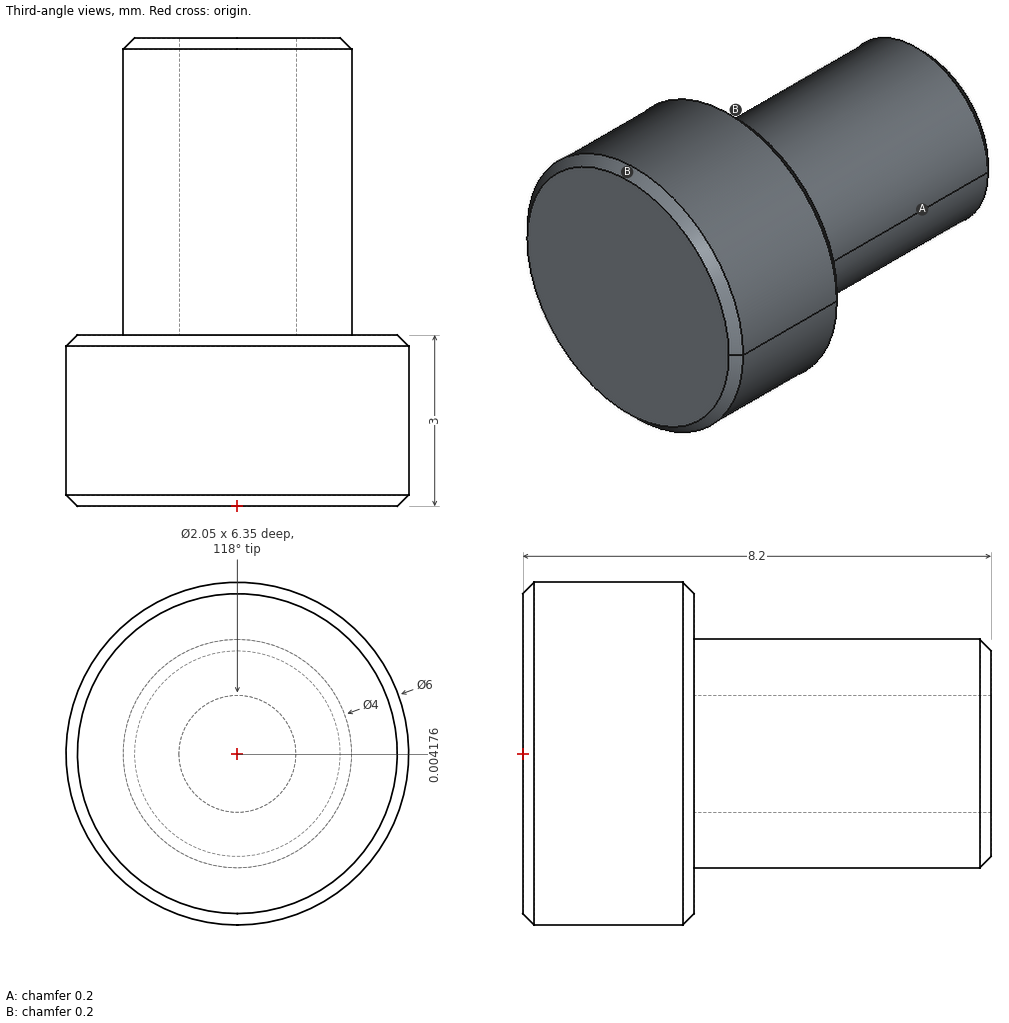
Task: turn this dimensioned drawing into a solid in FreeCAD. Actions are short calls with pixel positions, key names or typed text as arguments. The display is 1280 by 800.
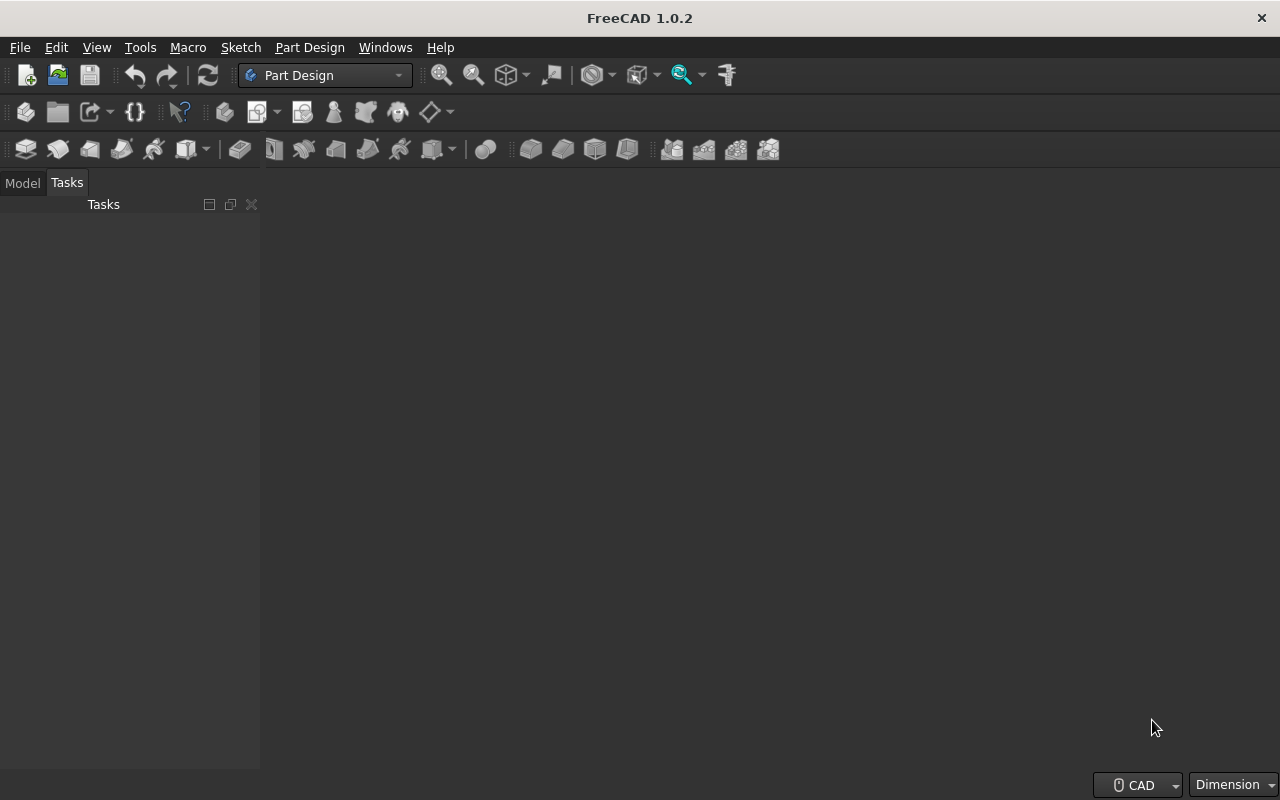
click(26, 76)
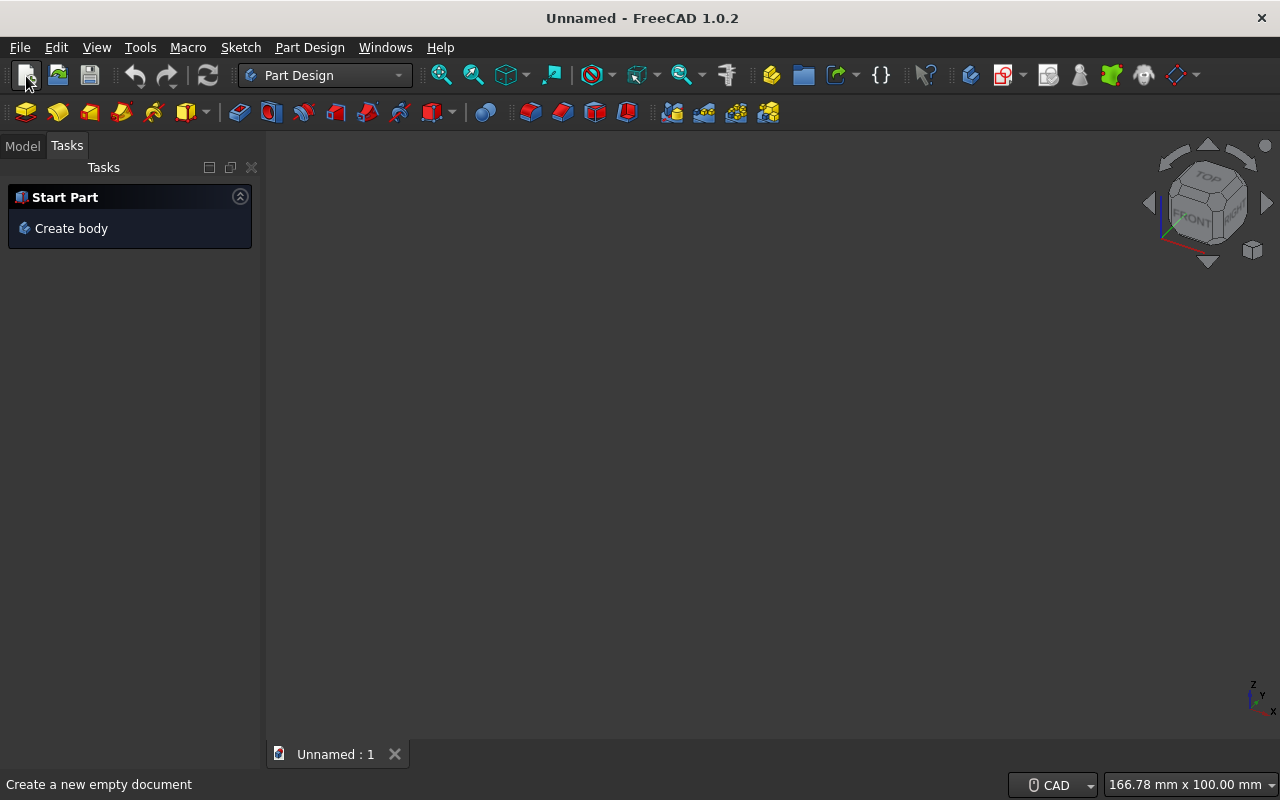
click(1004, 76)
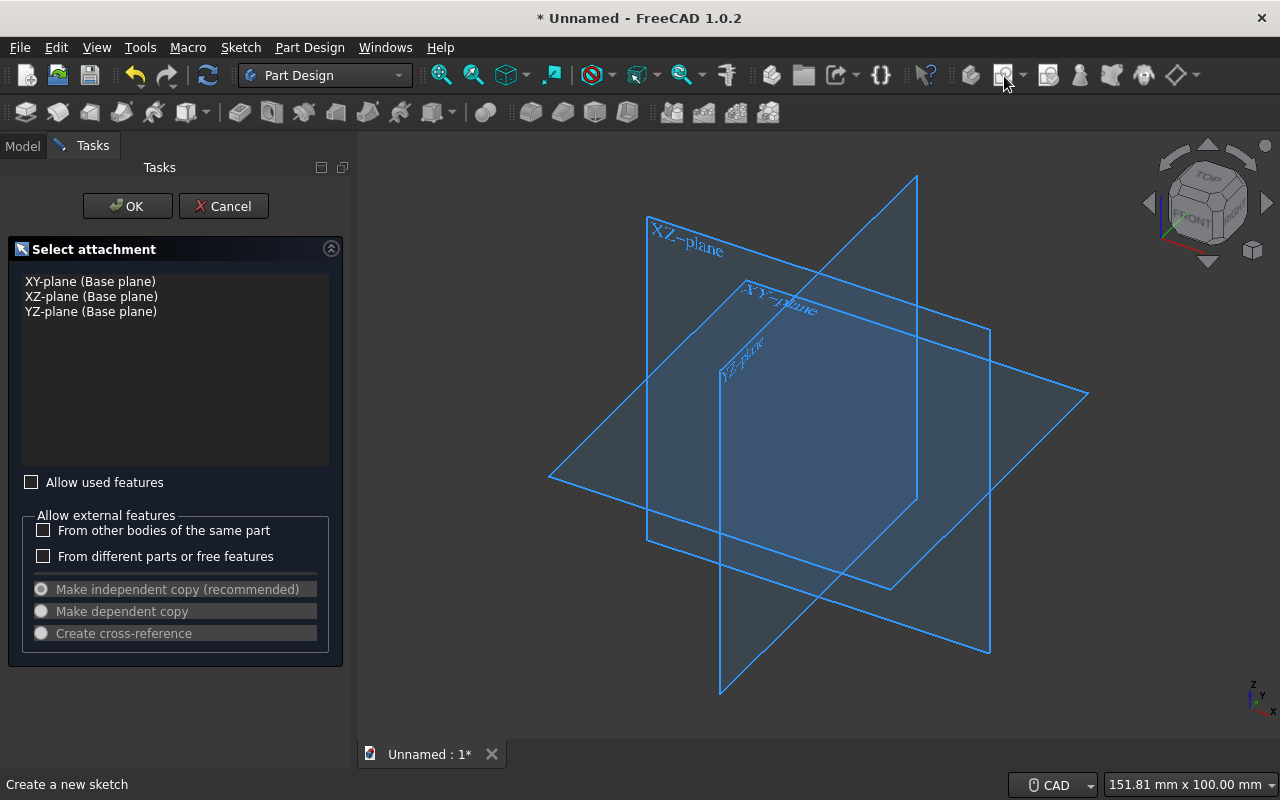
click(82, 296)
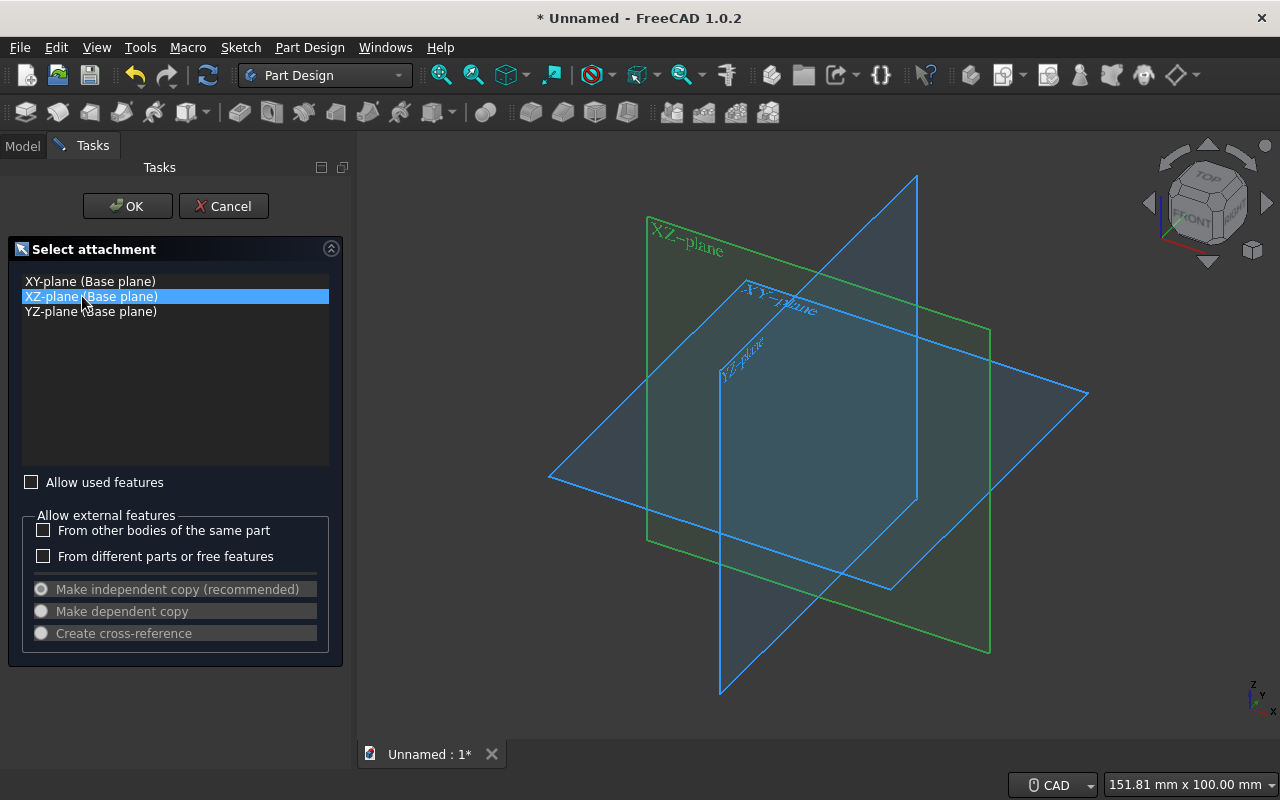
click(128, 206)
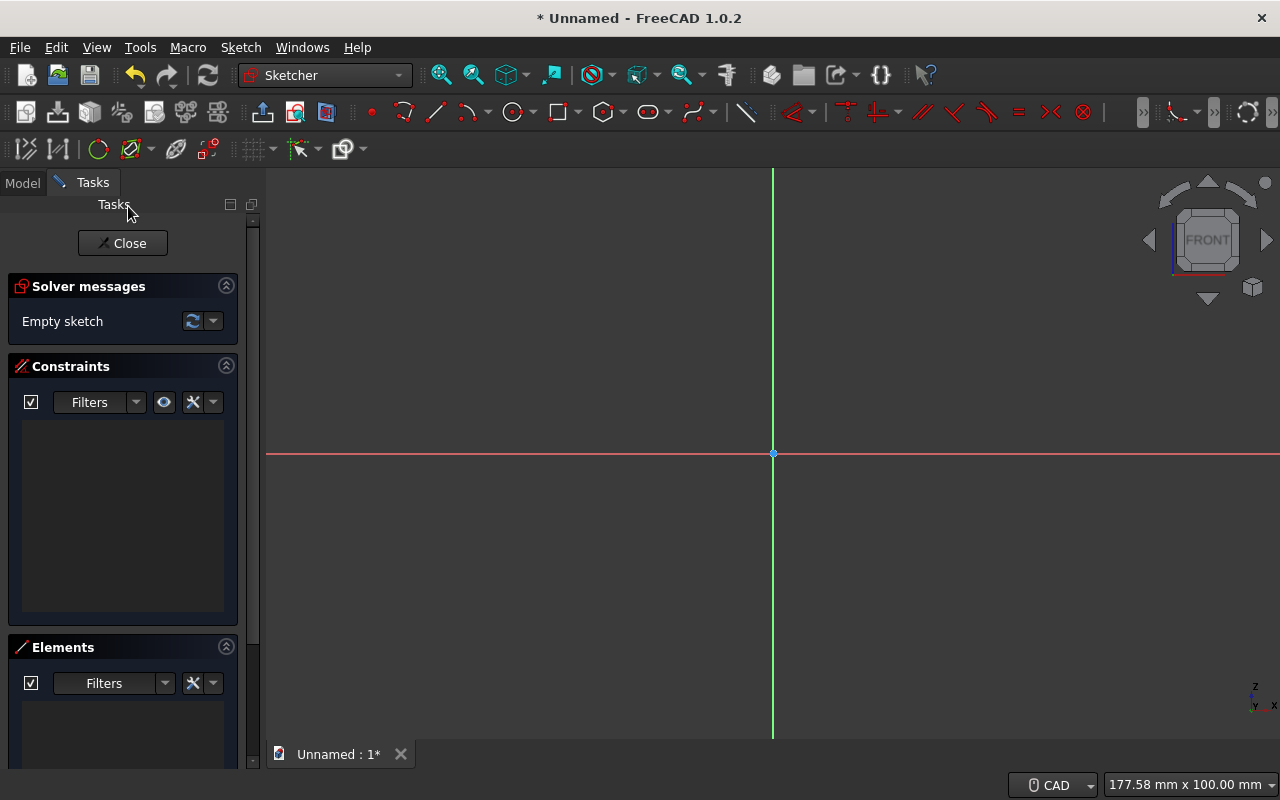
scroll(777, 454, up, 14)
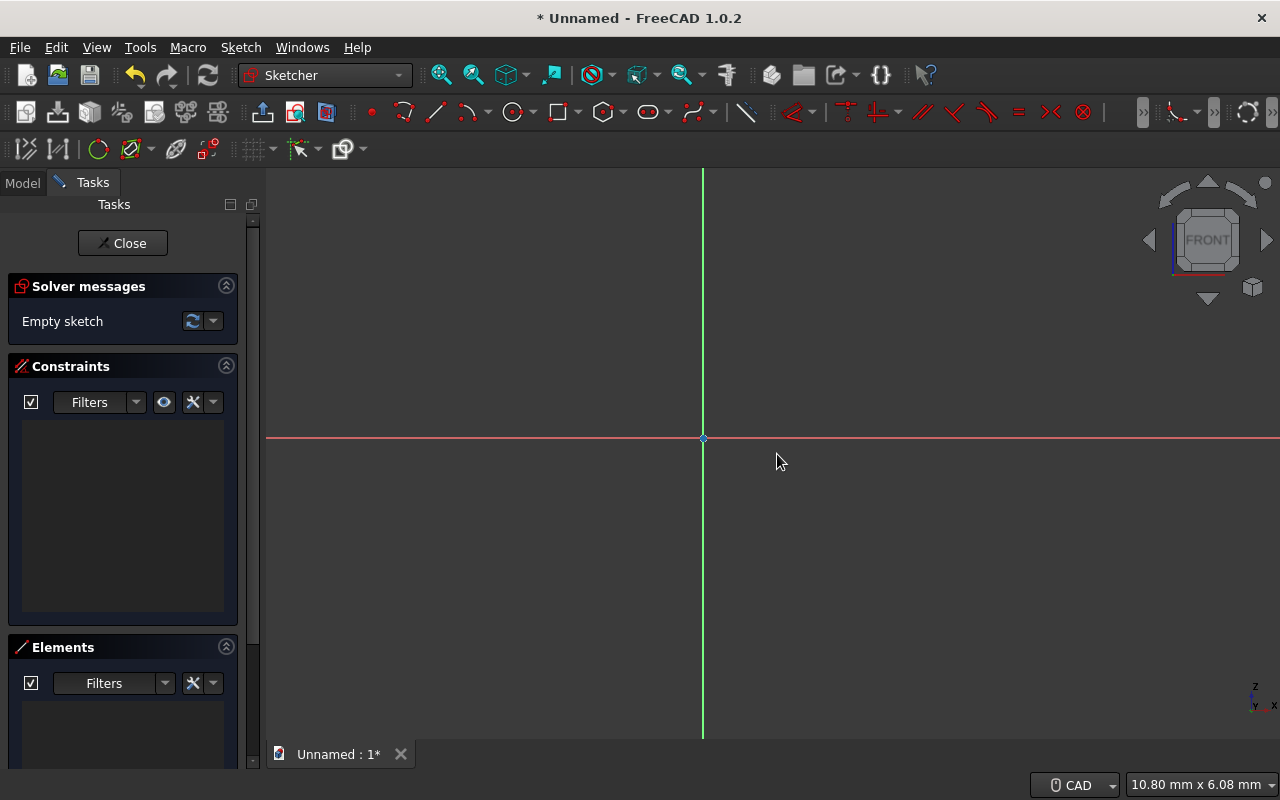
click(514, 112)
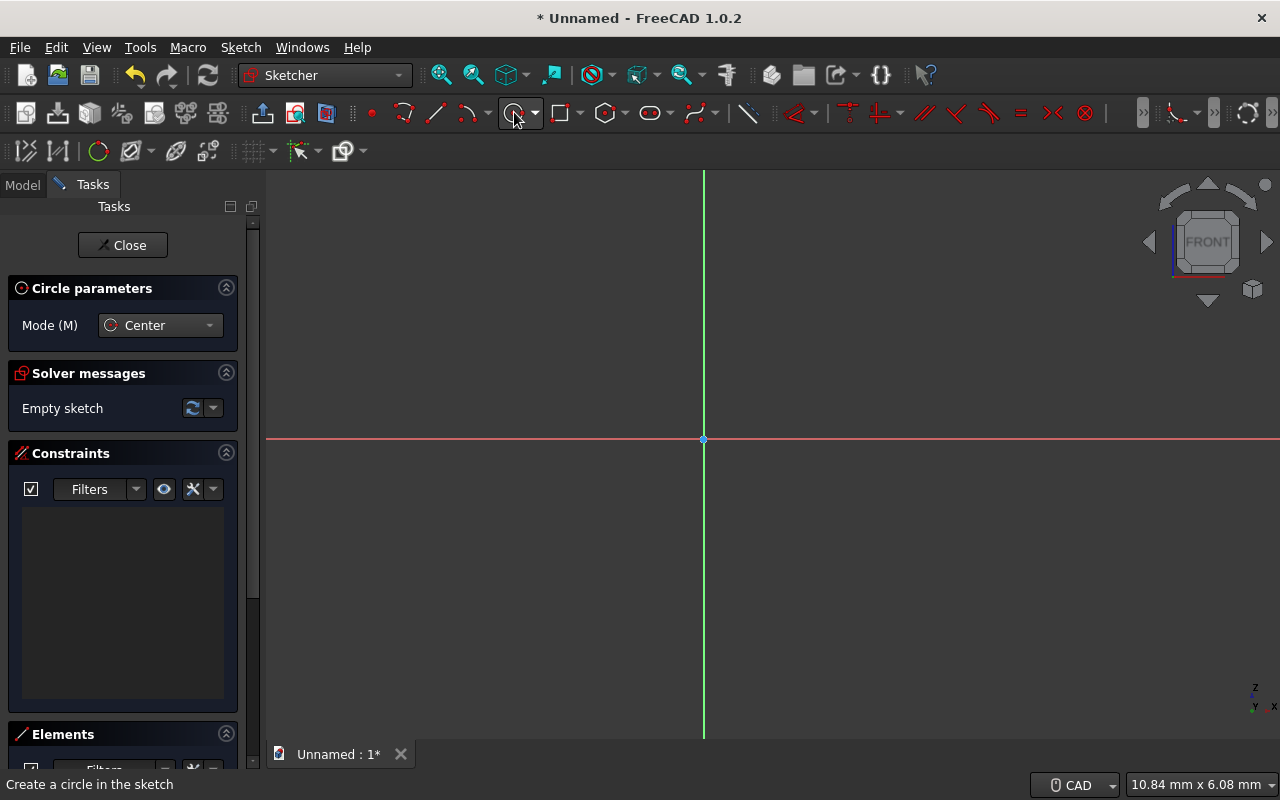
click(704, 439)
click(836, 307)
key(Escape)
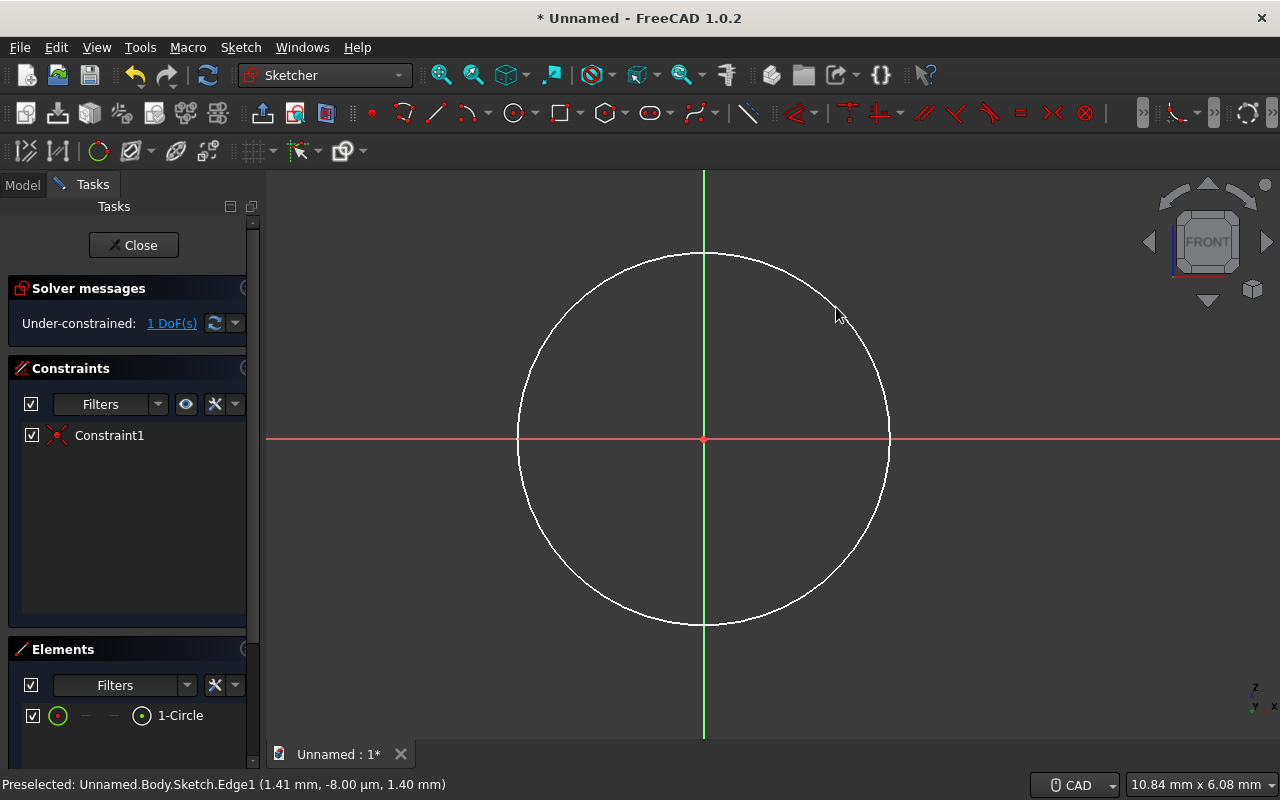
click(794, 114)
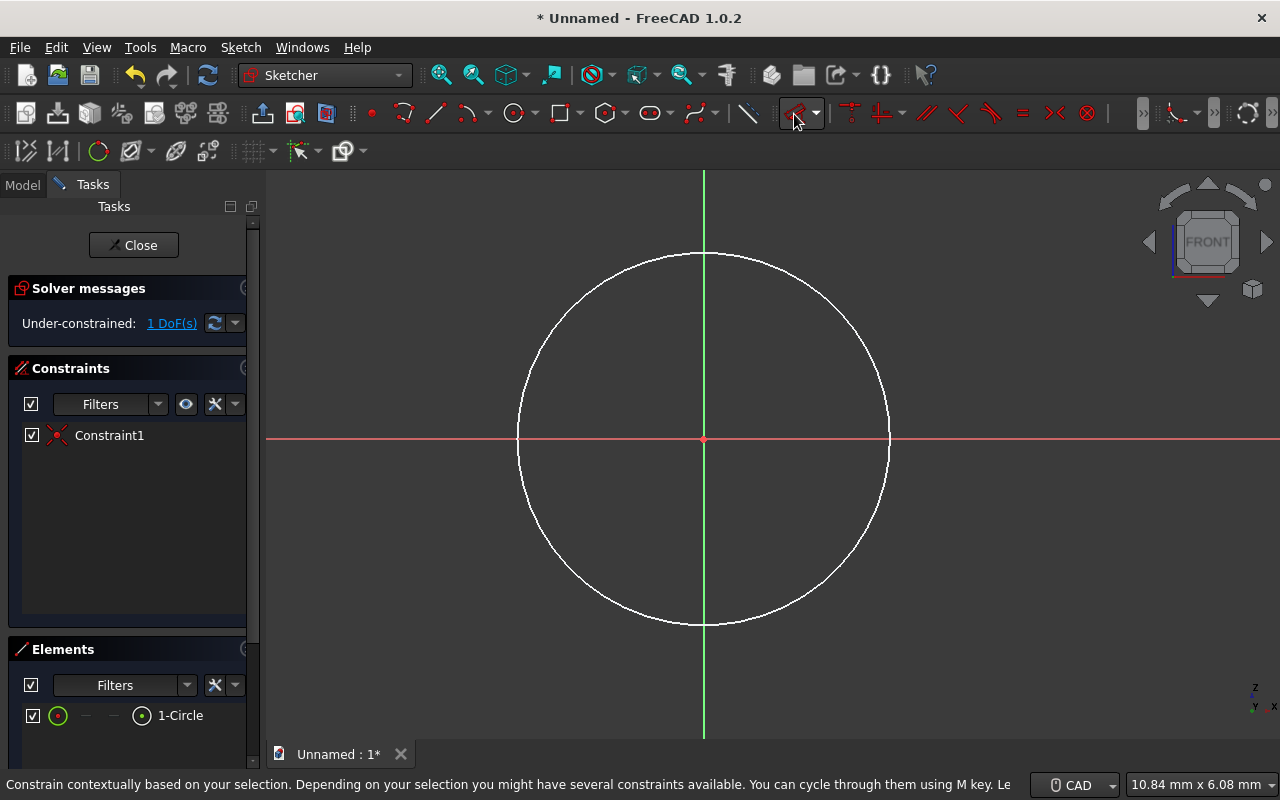
click(835, 307)
click(858, 284)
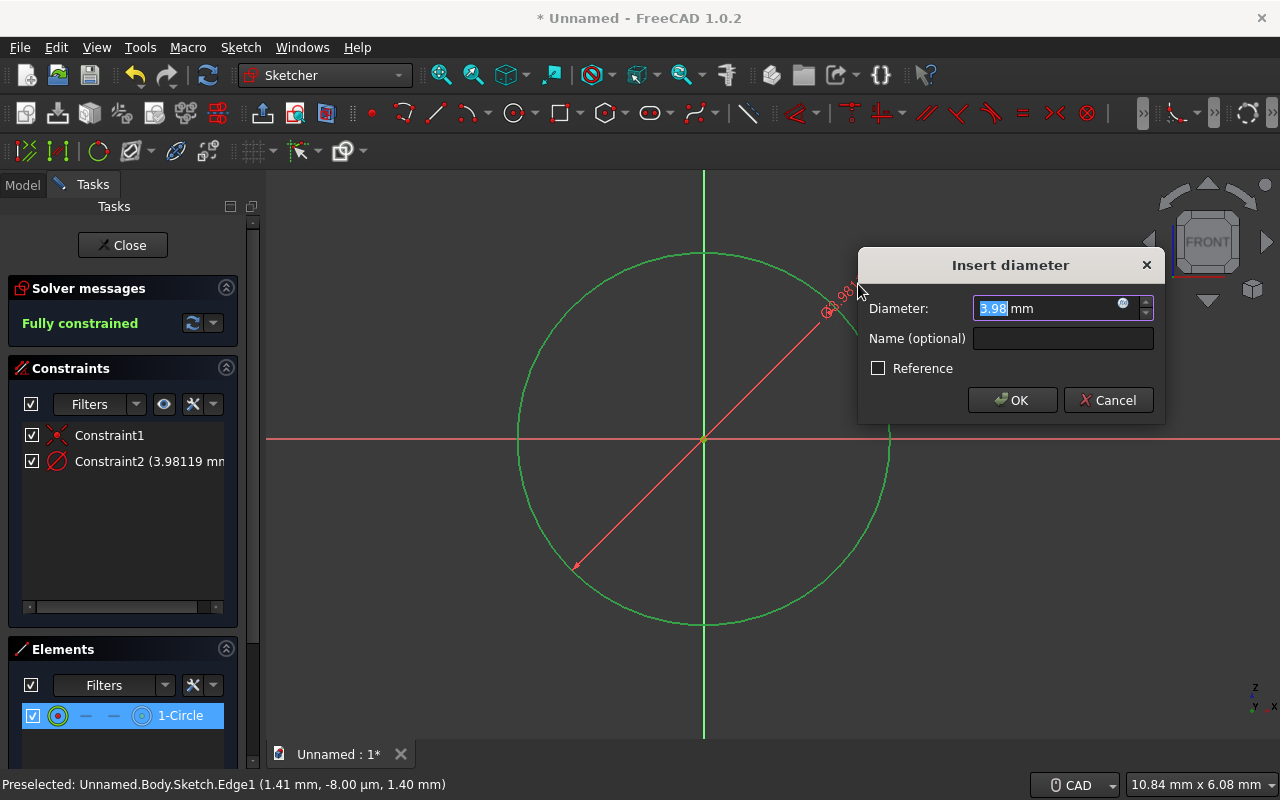
text(4)
key(Return)
key(Escape)